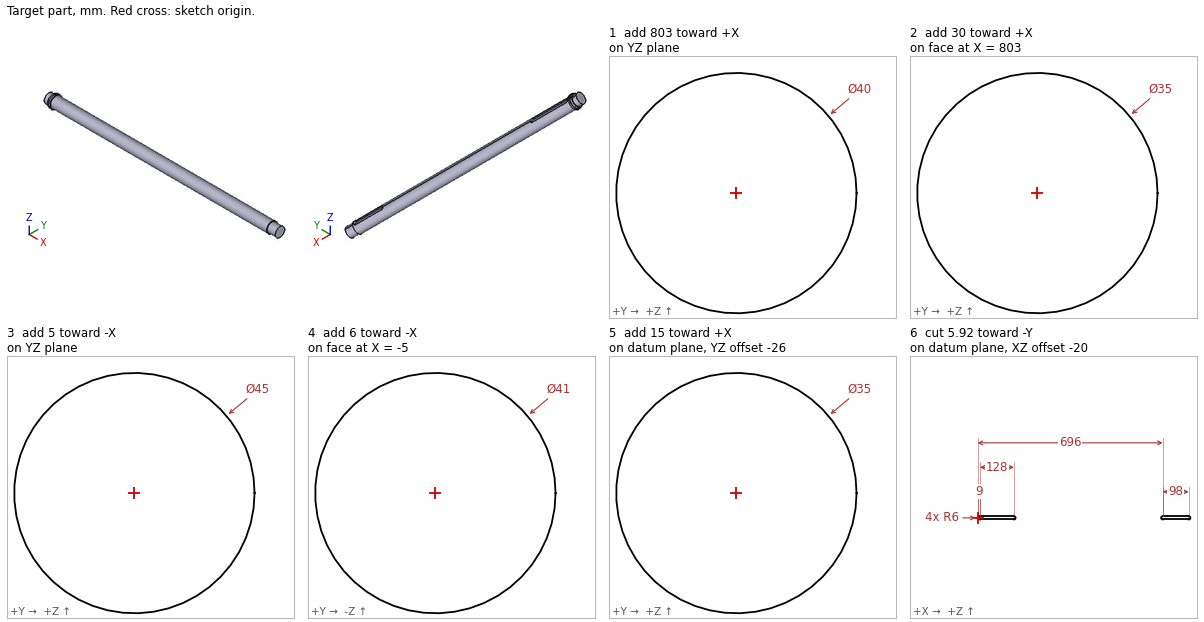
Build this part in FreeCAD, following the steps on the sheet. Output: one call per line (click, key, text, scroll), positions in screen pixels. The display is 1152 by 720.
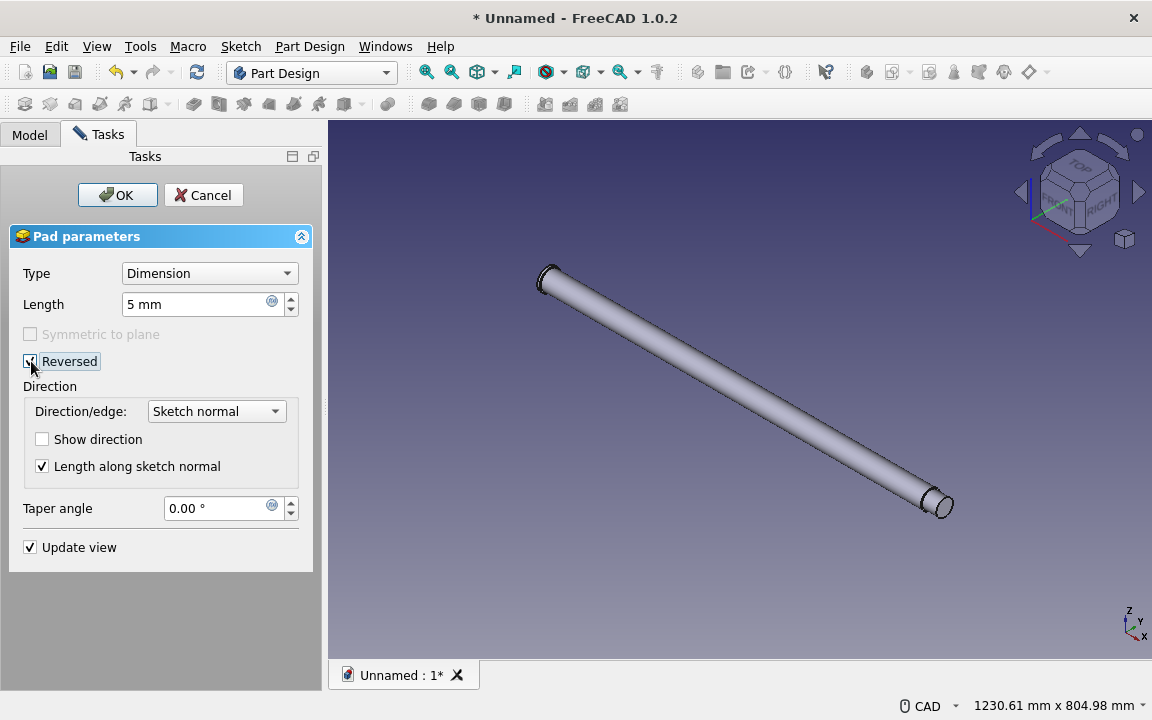
click(118, 195)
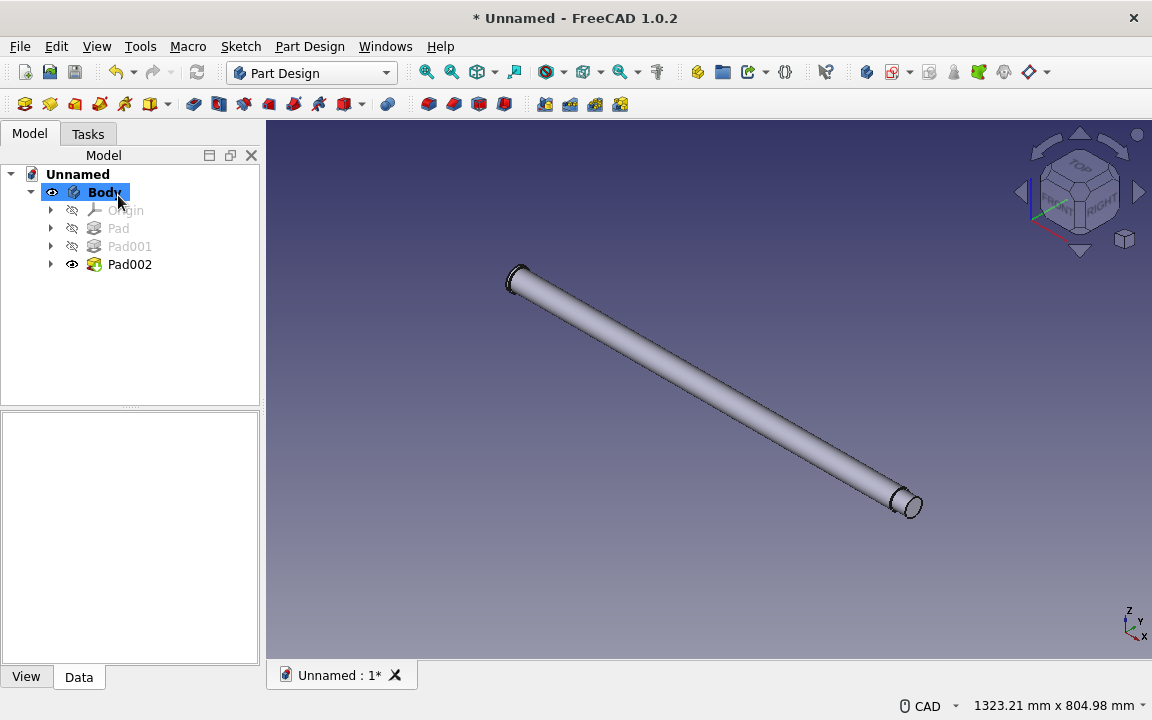
key(6)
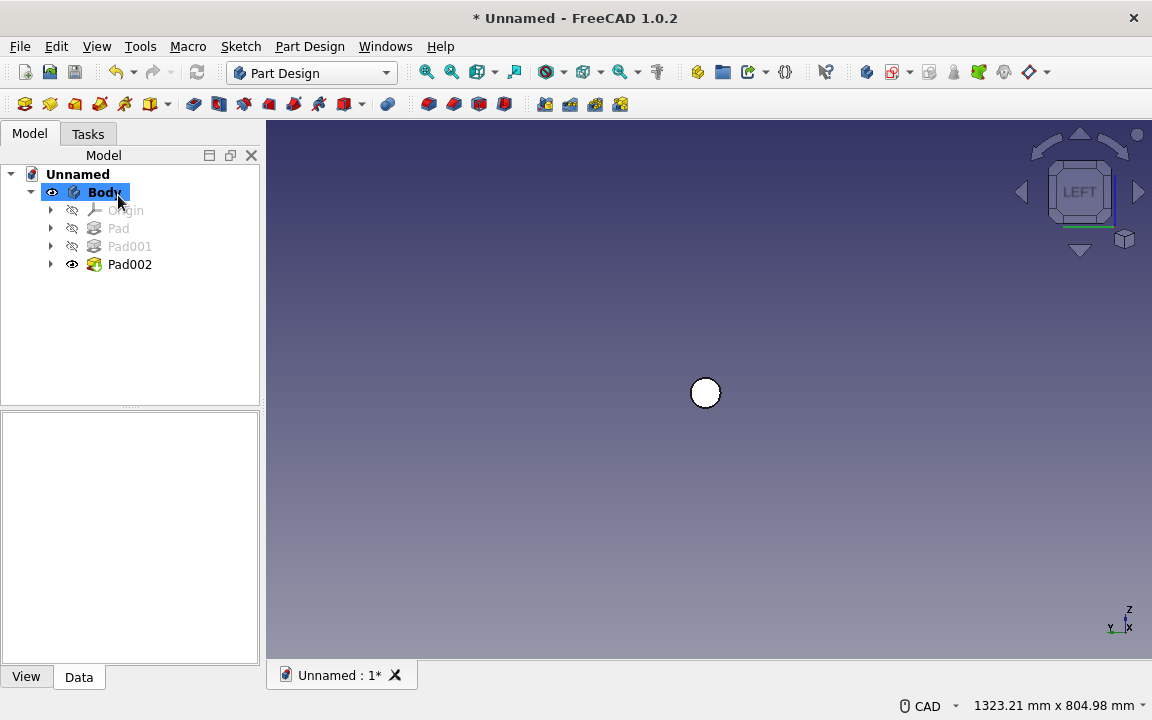
click(427, 72)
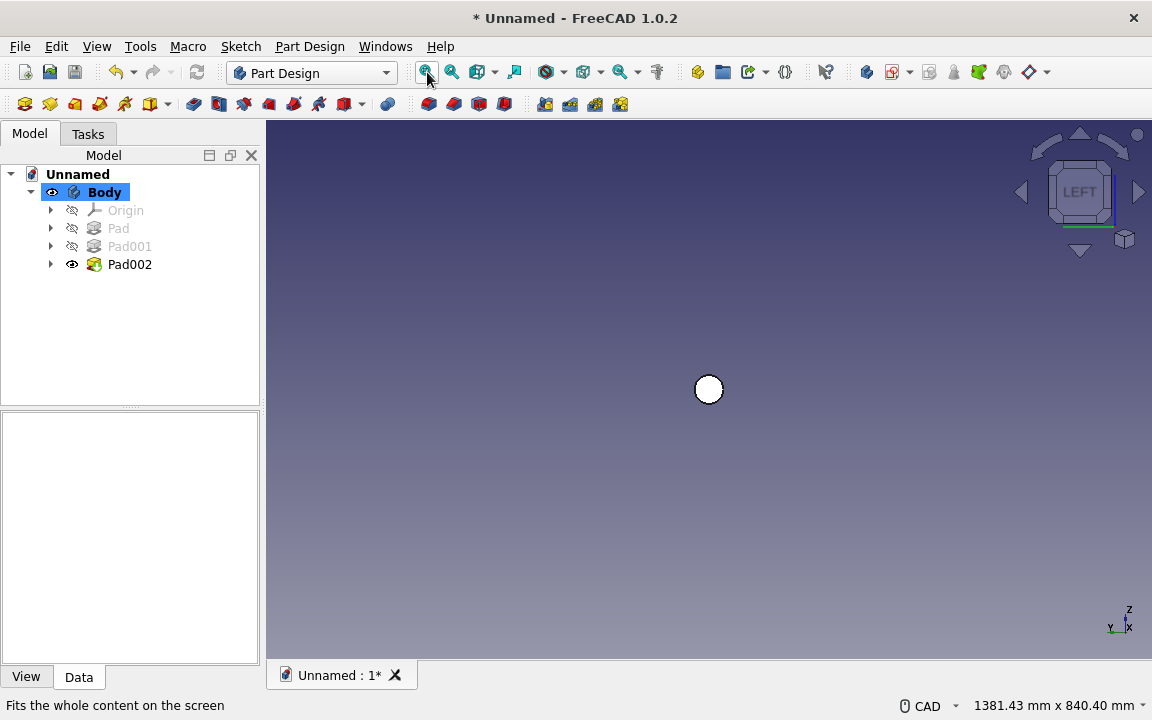
click(709, 388)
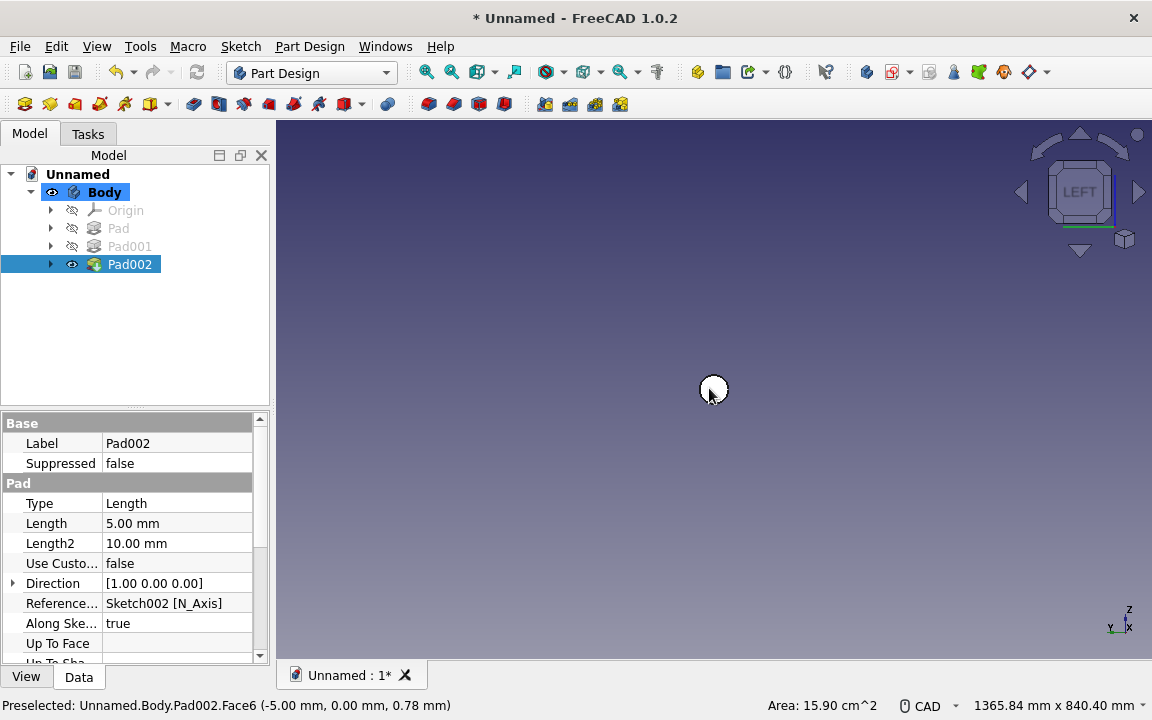
click(892, 72)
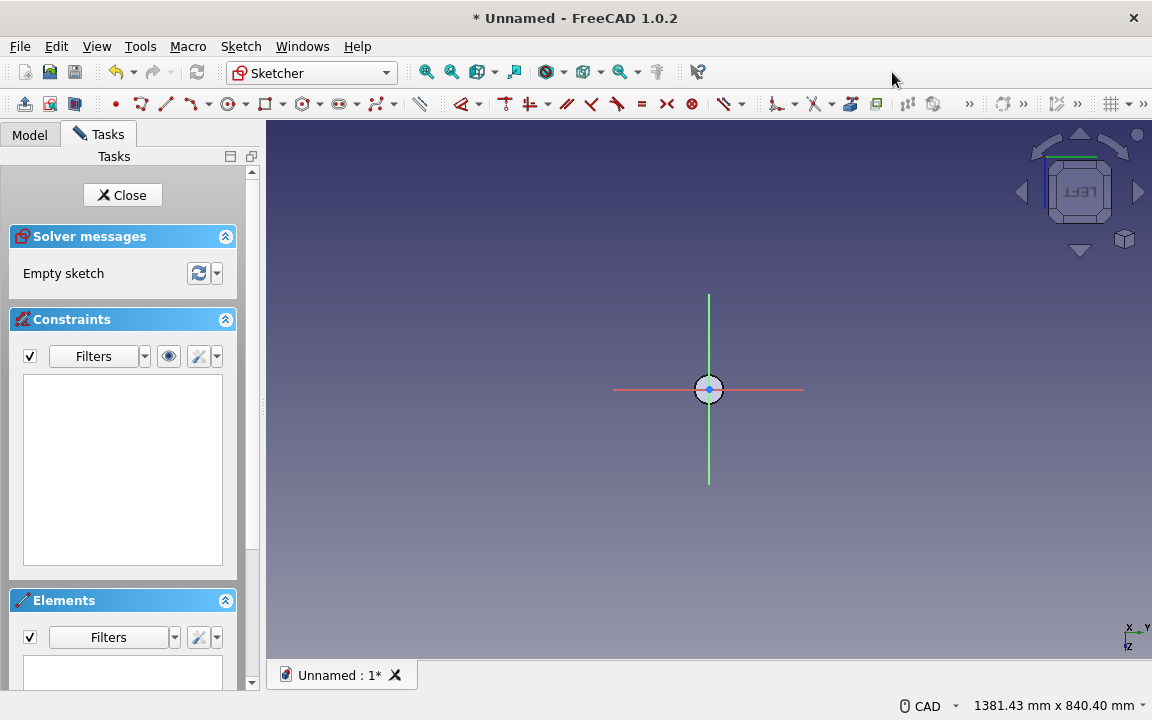
scroll(714, 390, up, 13)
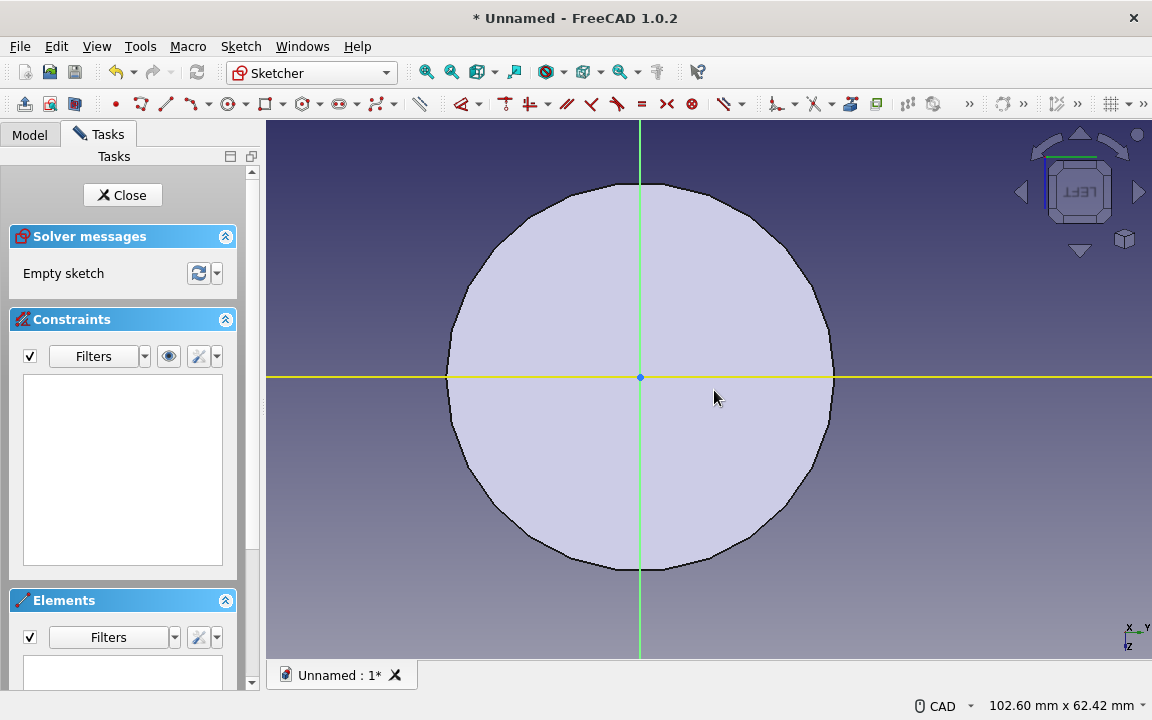
click(228, 104)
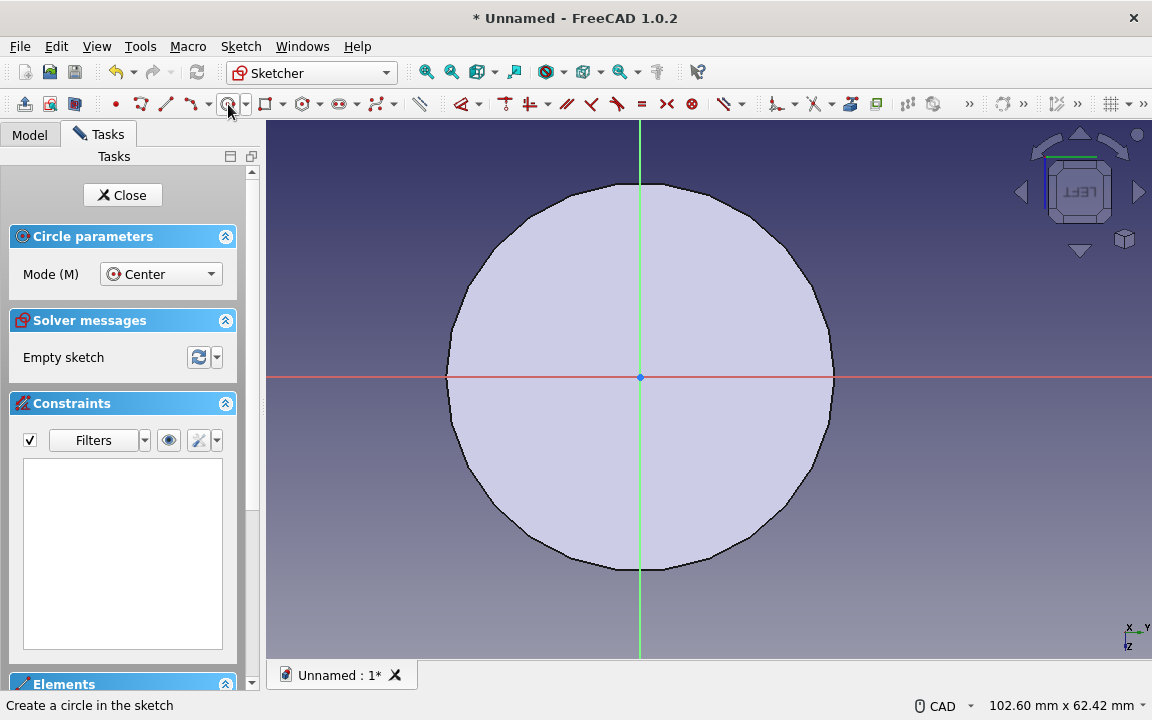
click(640, 377)
move(766, 252)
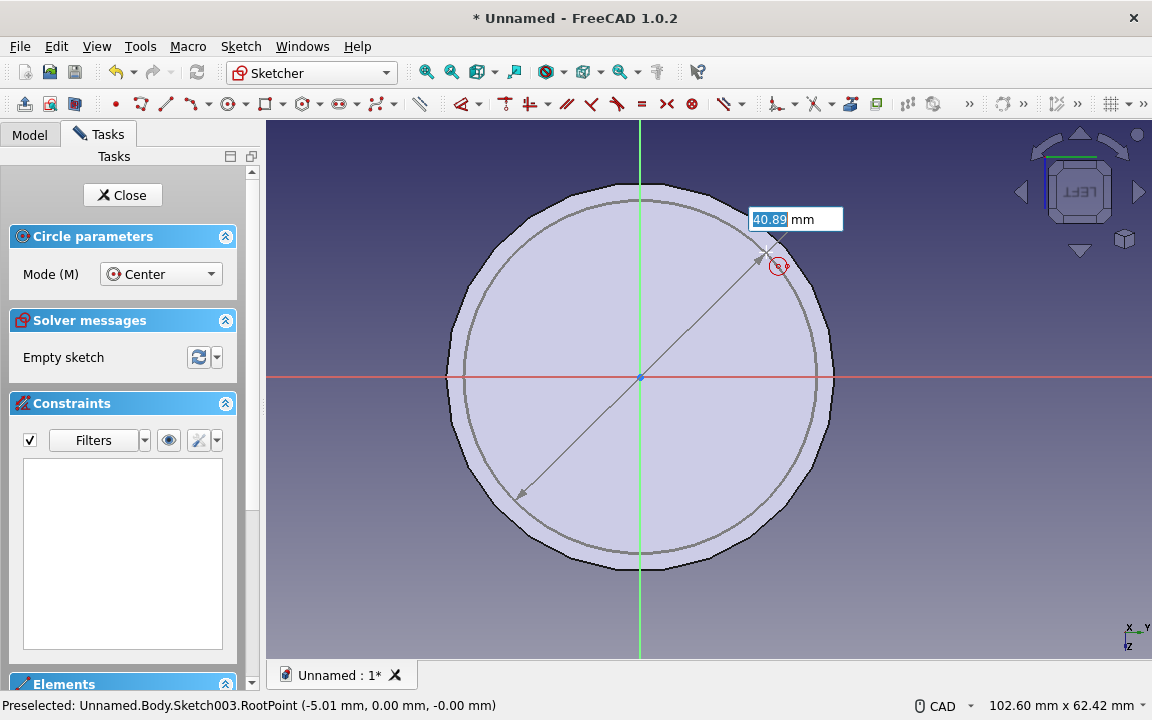
text(41)
key(Return)
key(Escape)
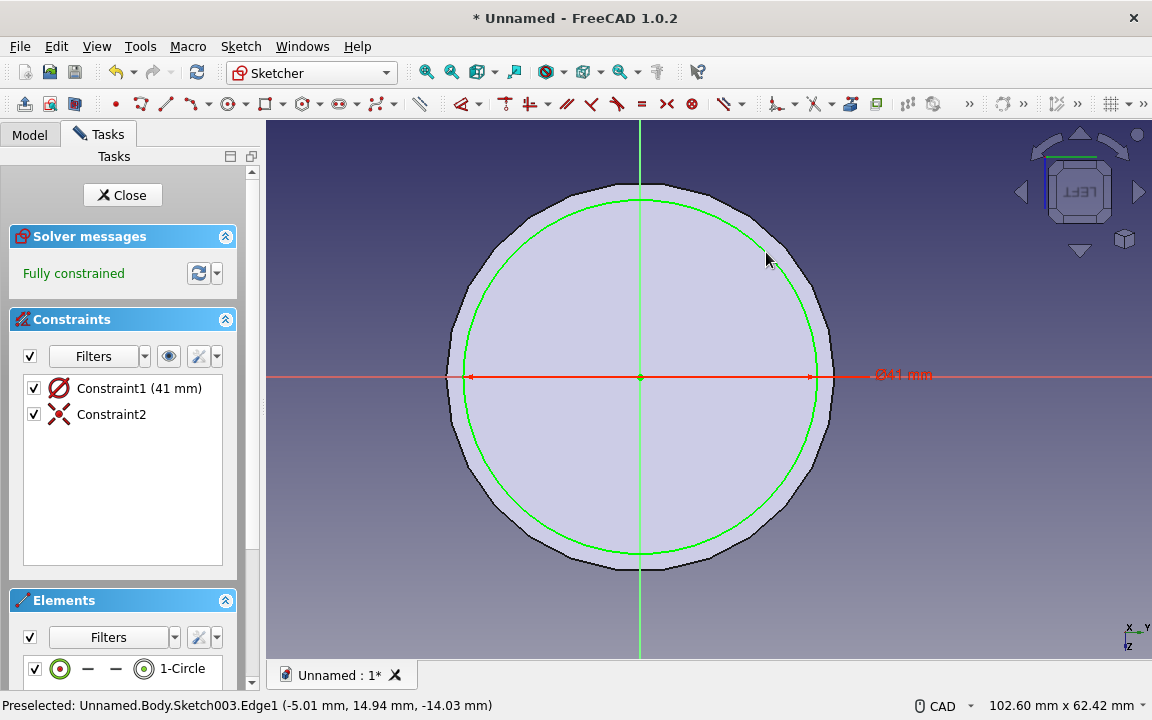
click(123, 195)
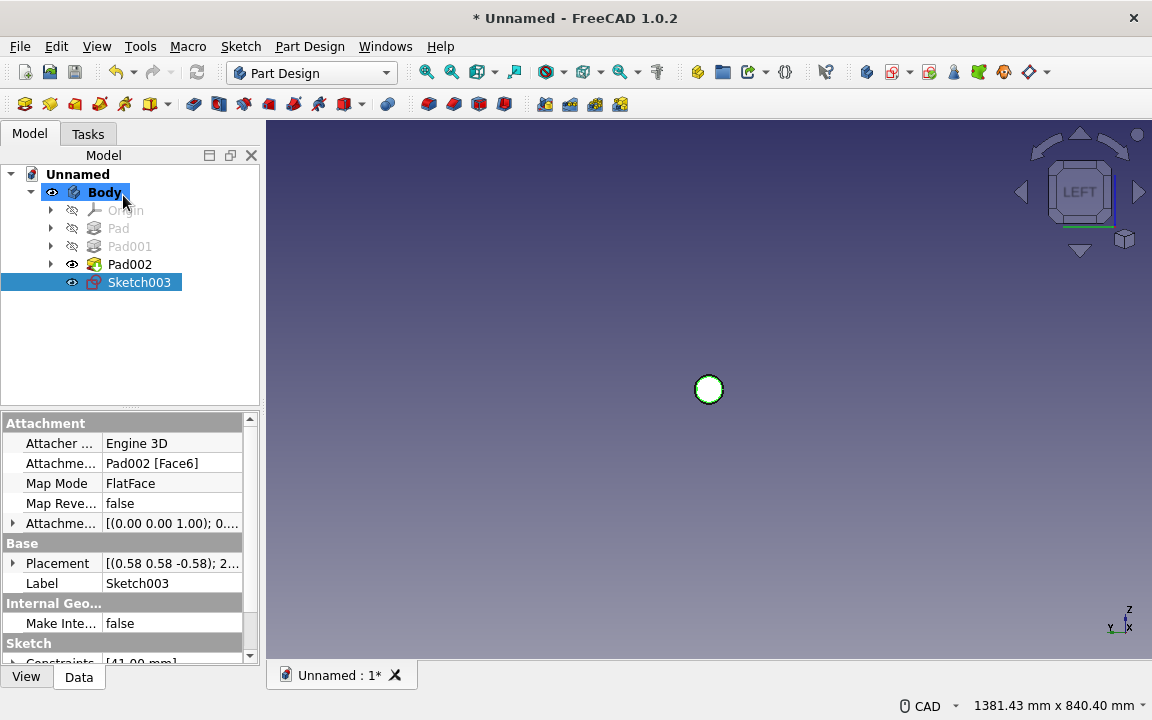
click(25, 104)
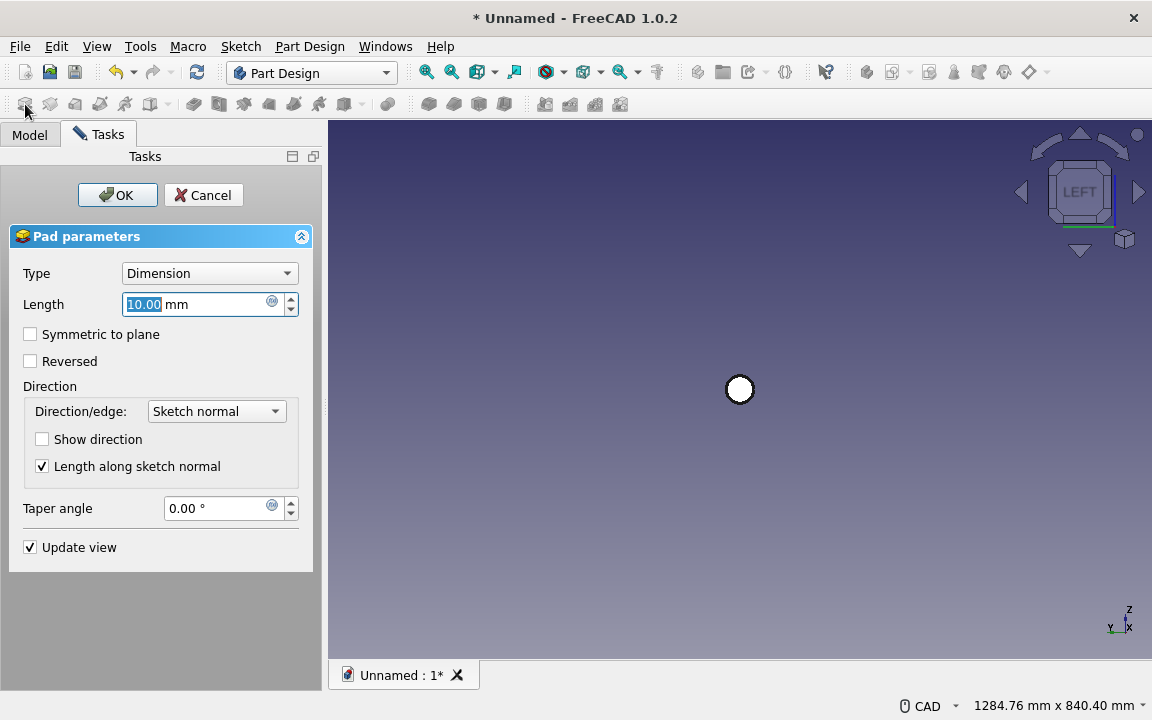
text(6)
key(Tab)